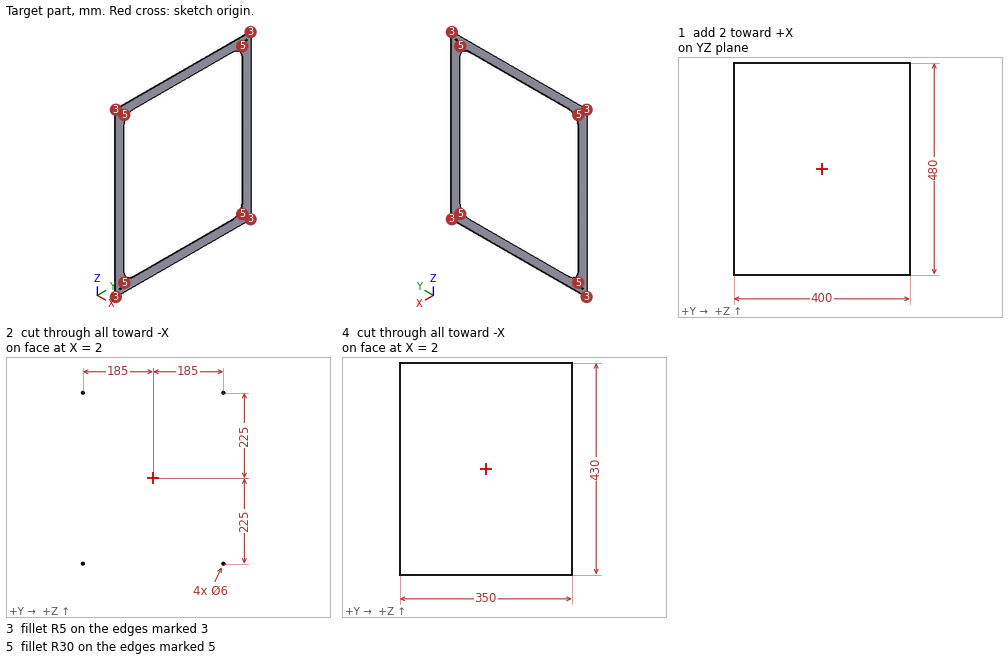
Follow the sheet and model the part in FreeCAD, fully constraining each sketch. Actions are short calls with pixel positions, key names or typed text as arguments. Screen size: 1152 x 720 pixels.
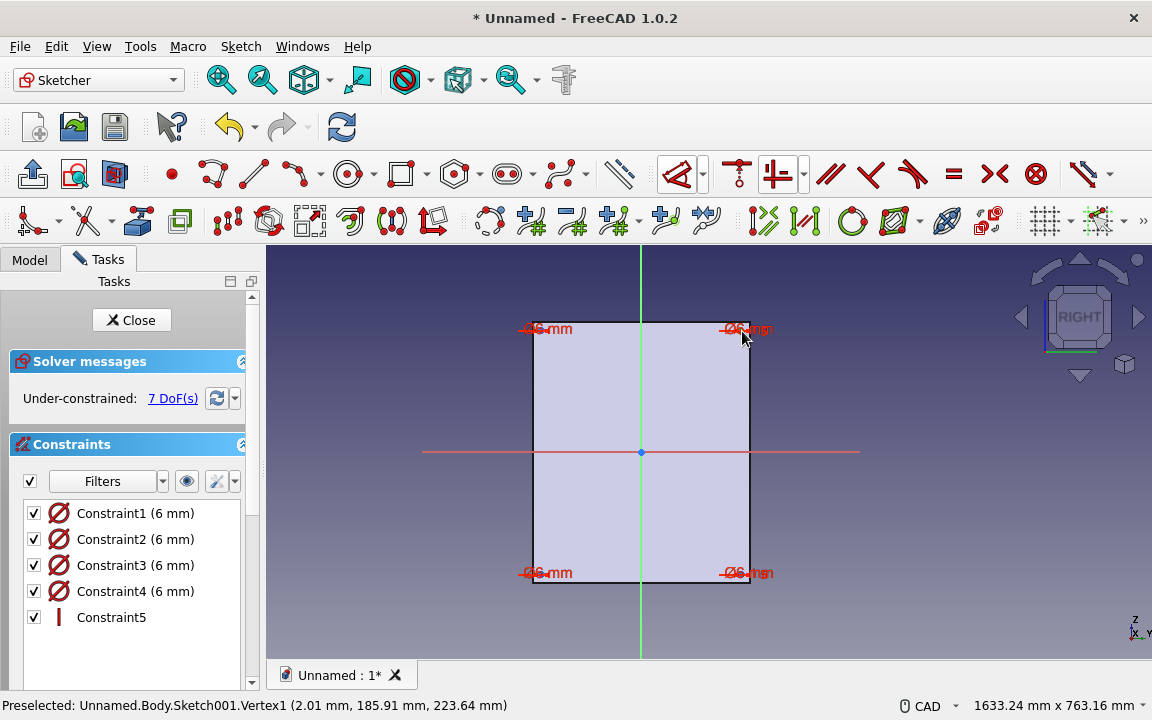
click(541, 331)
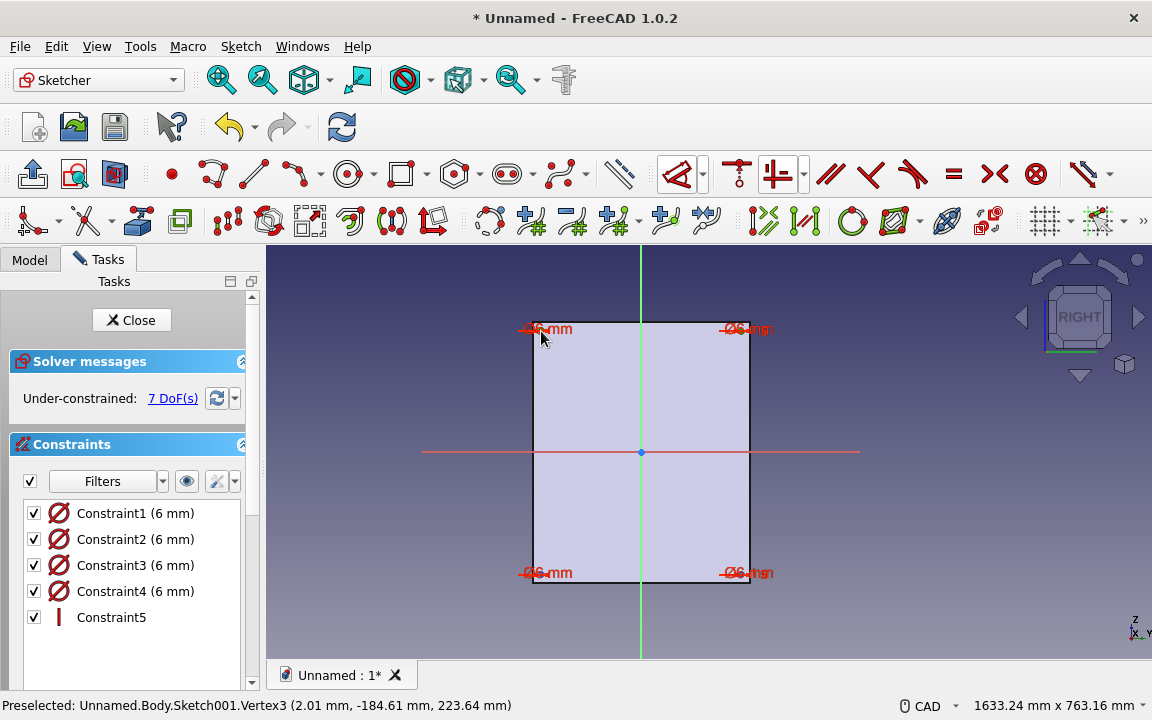
click(804, 174)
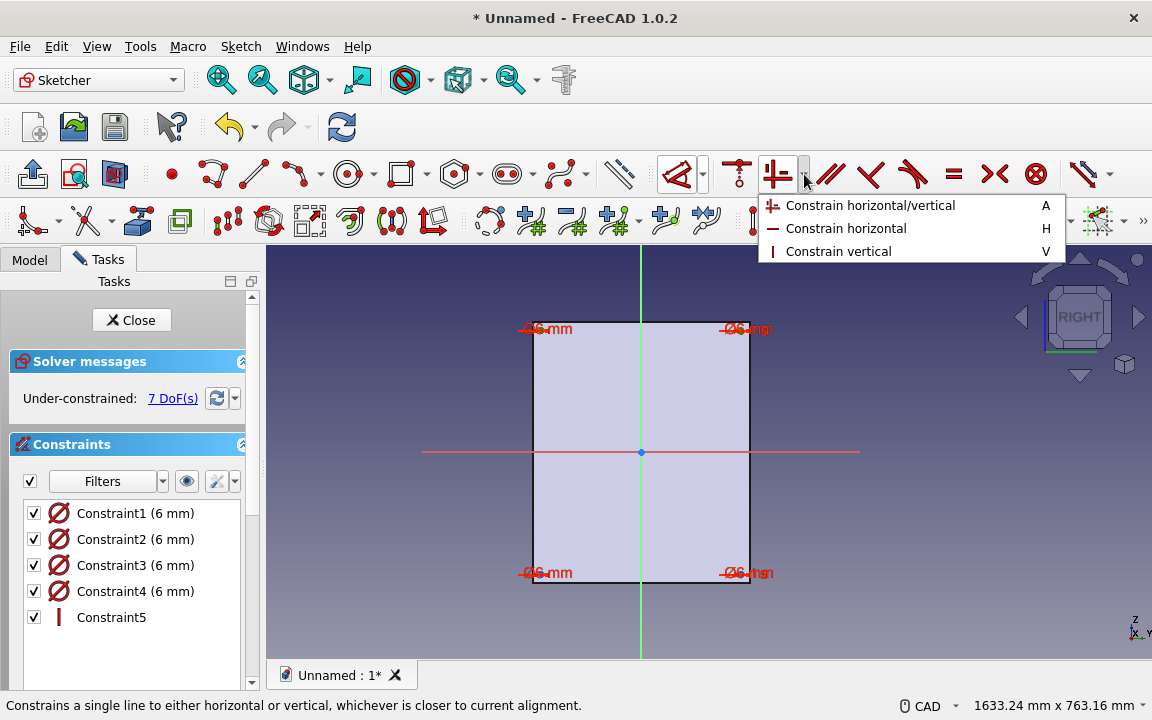
click(912, 228)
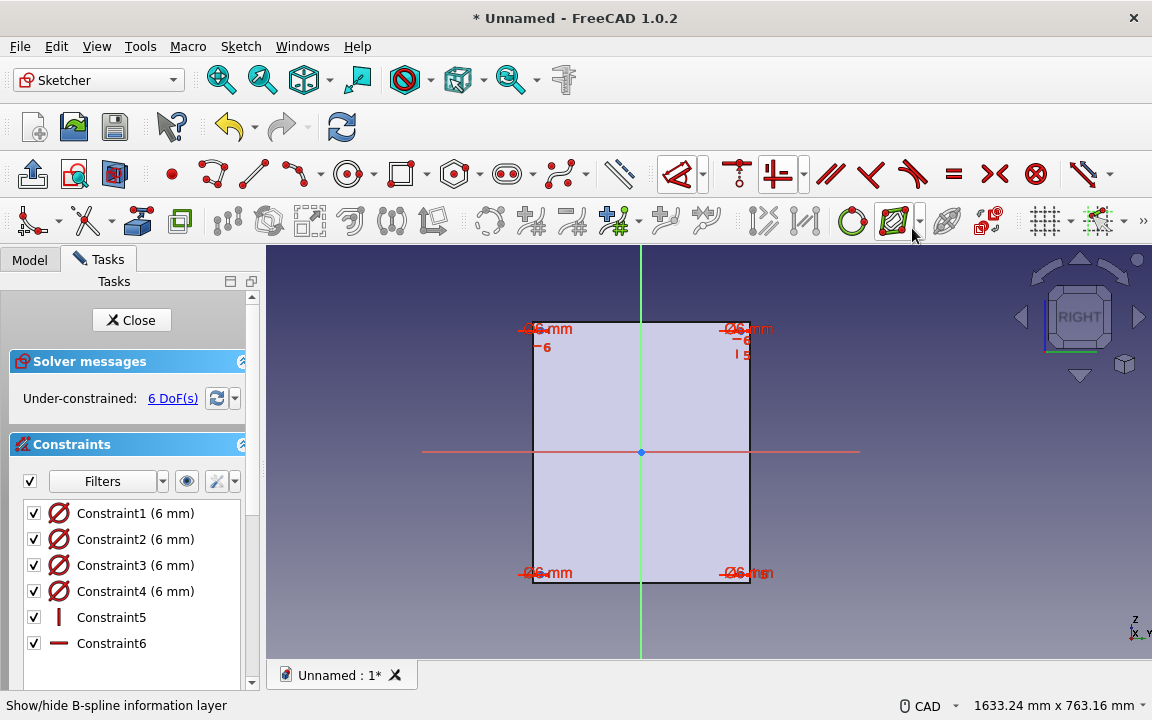
click(541, 331)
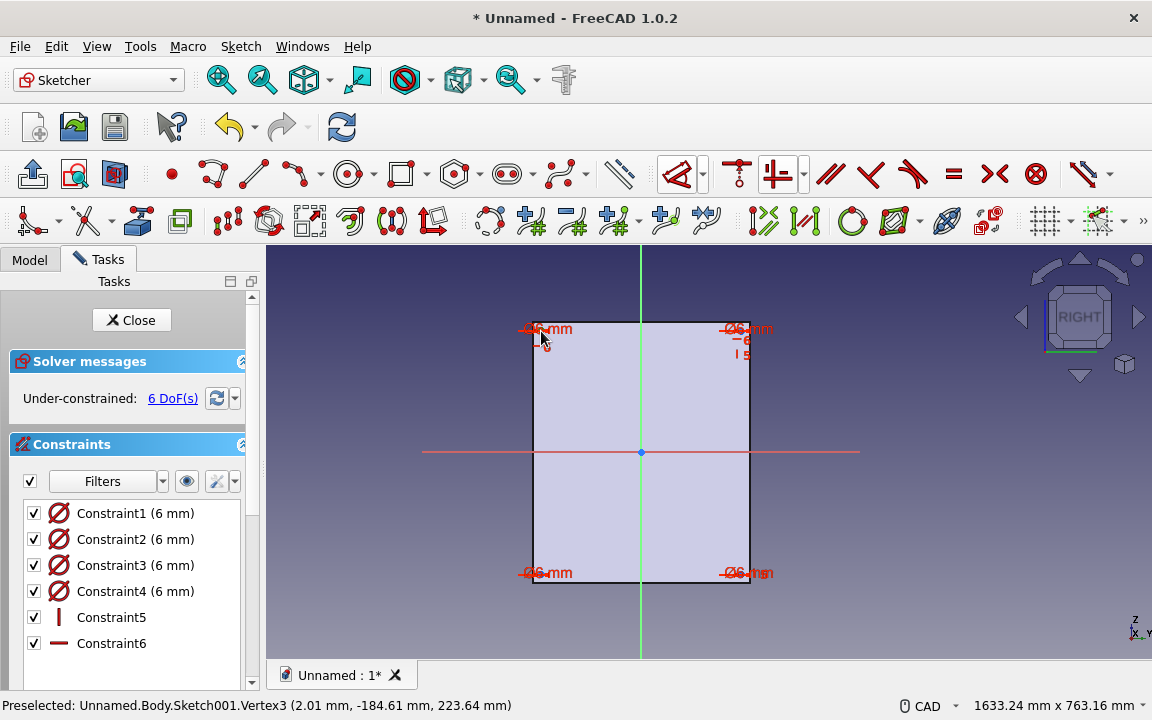
click(541, 575)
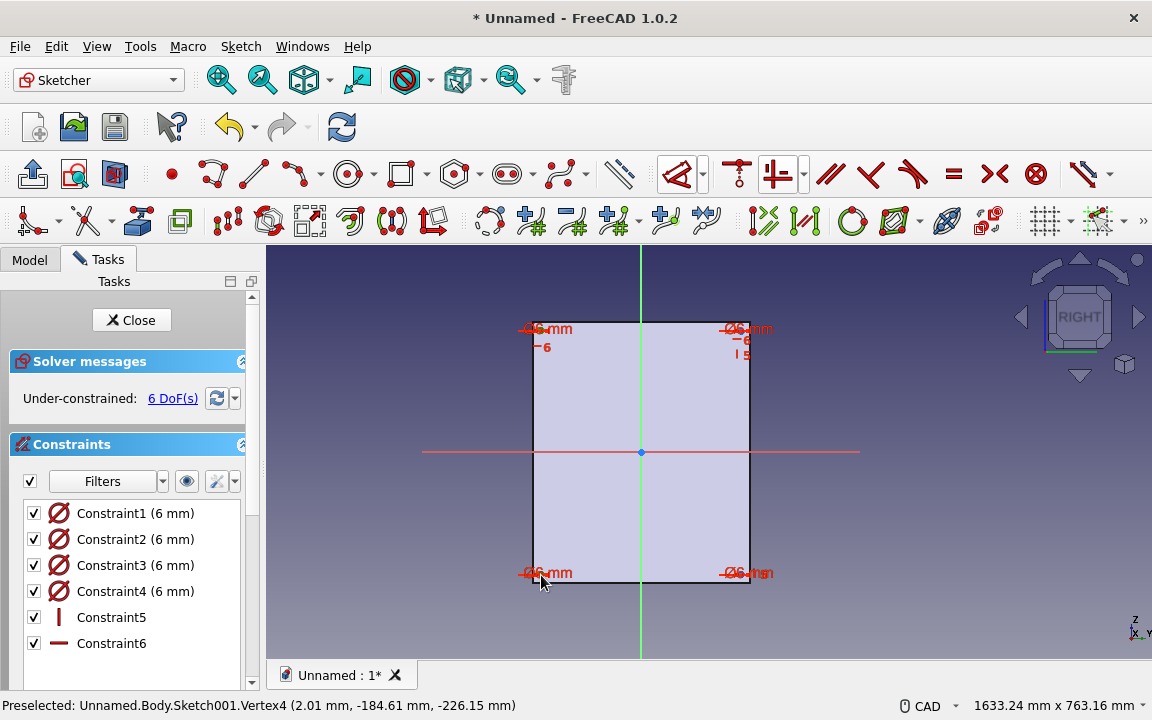
key(v)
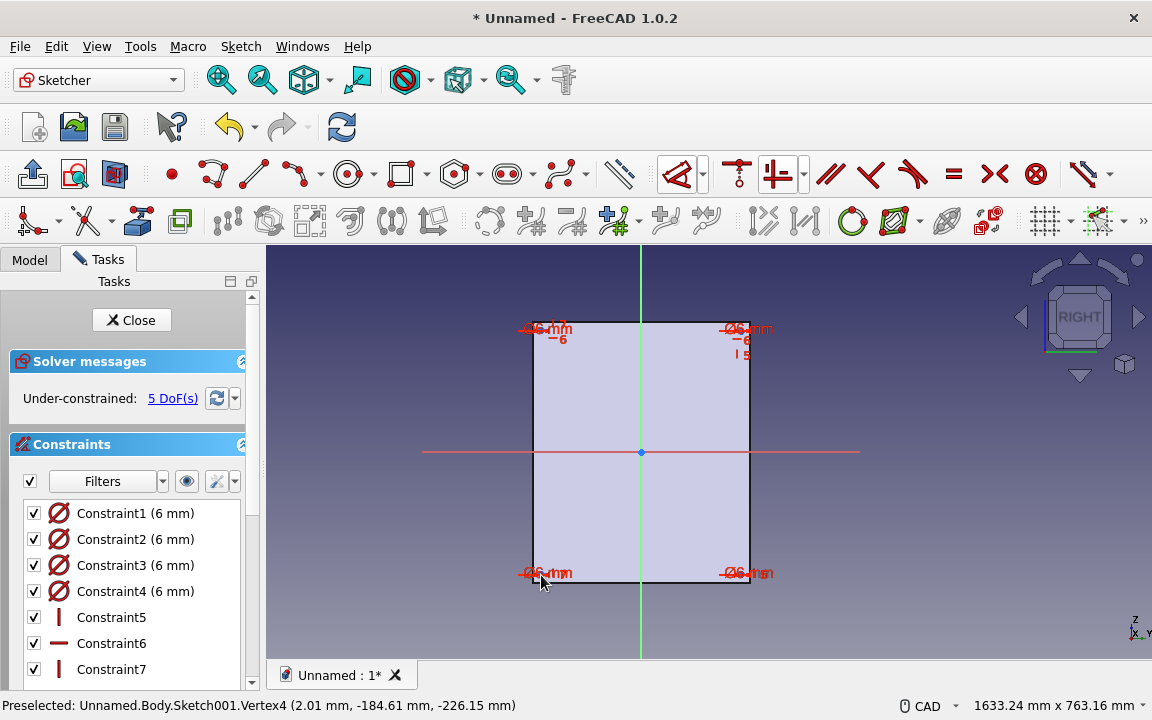
click(742, 575)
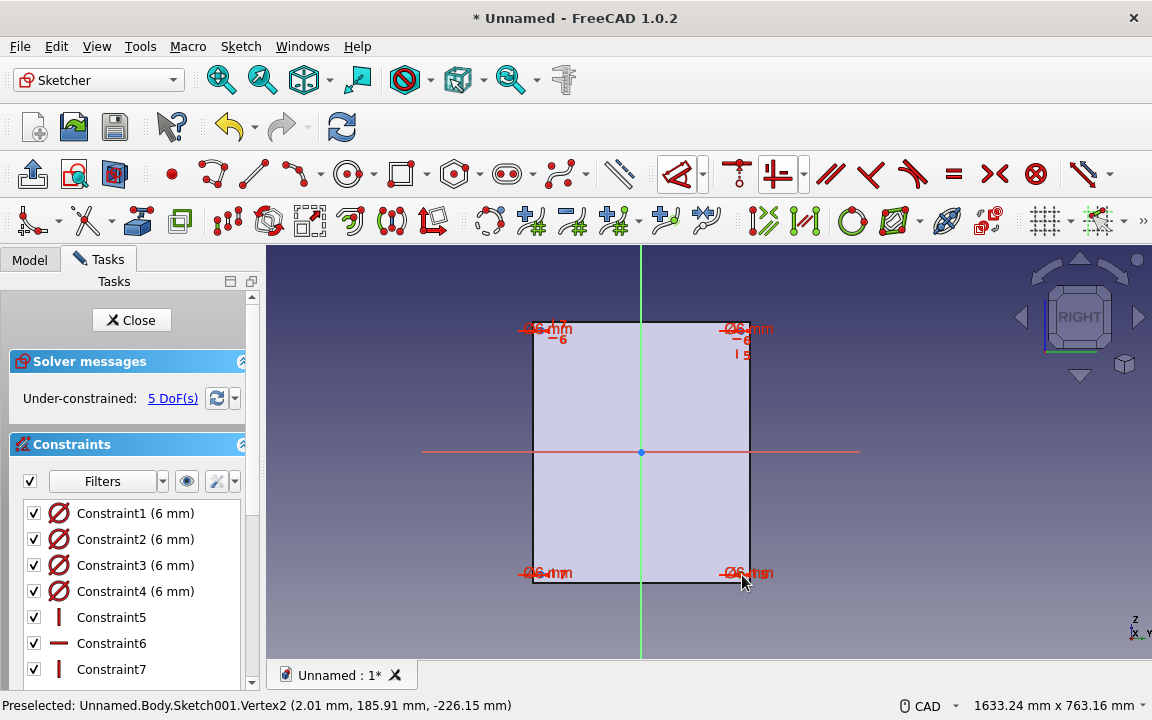
click(541, 575)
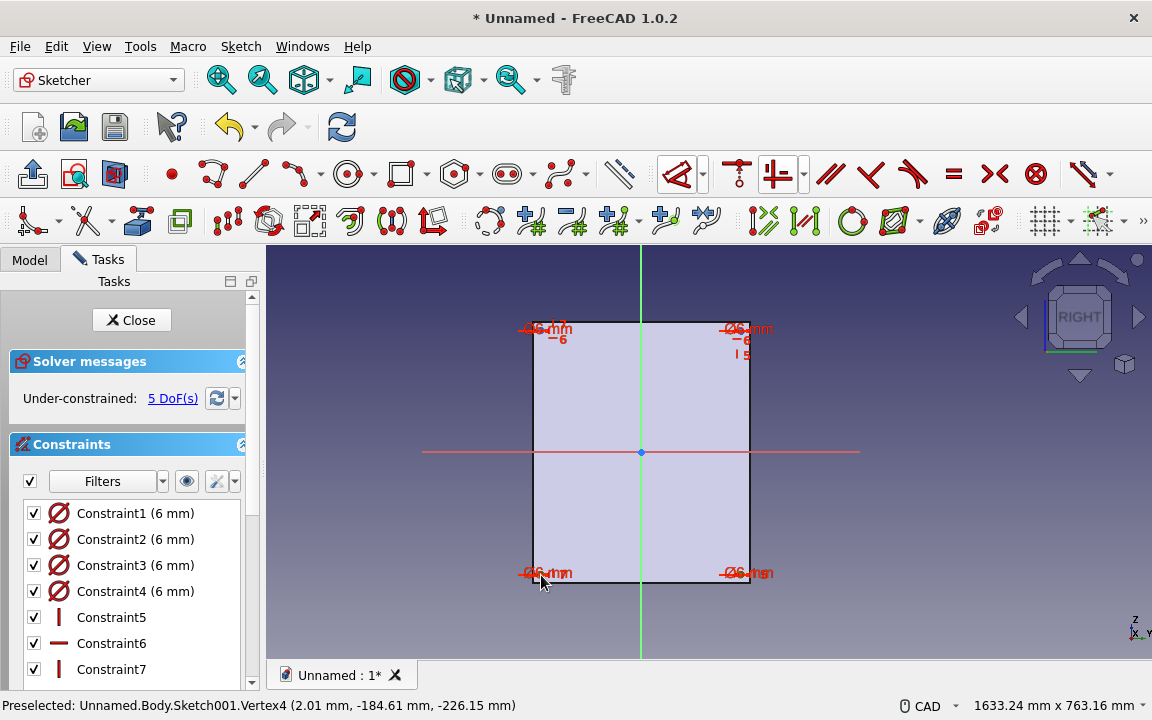
key(h)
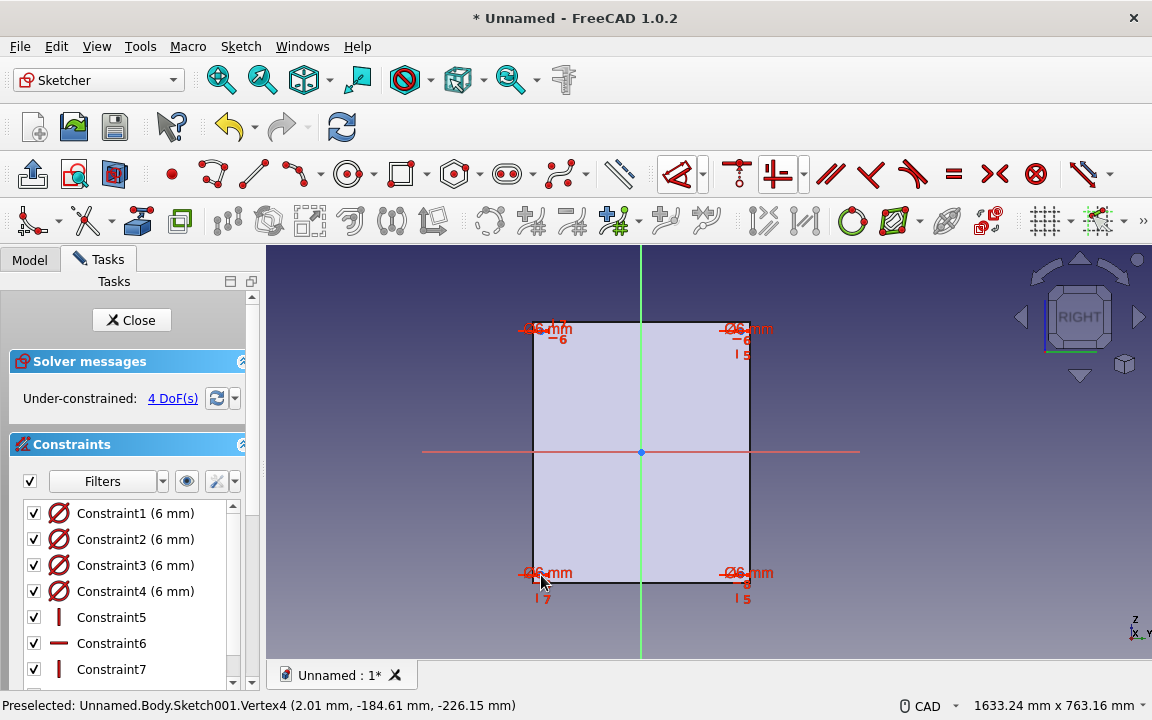
key(d)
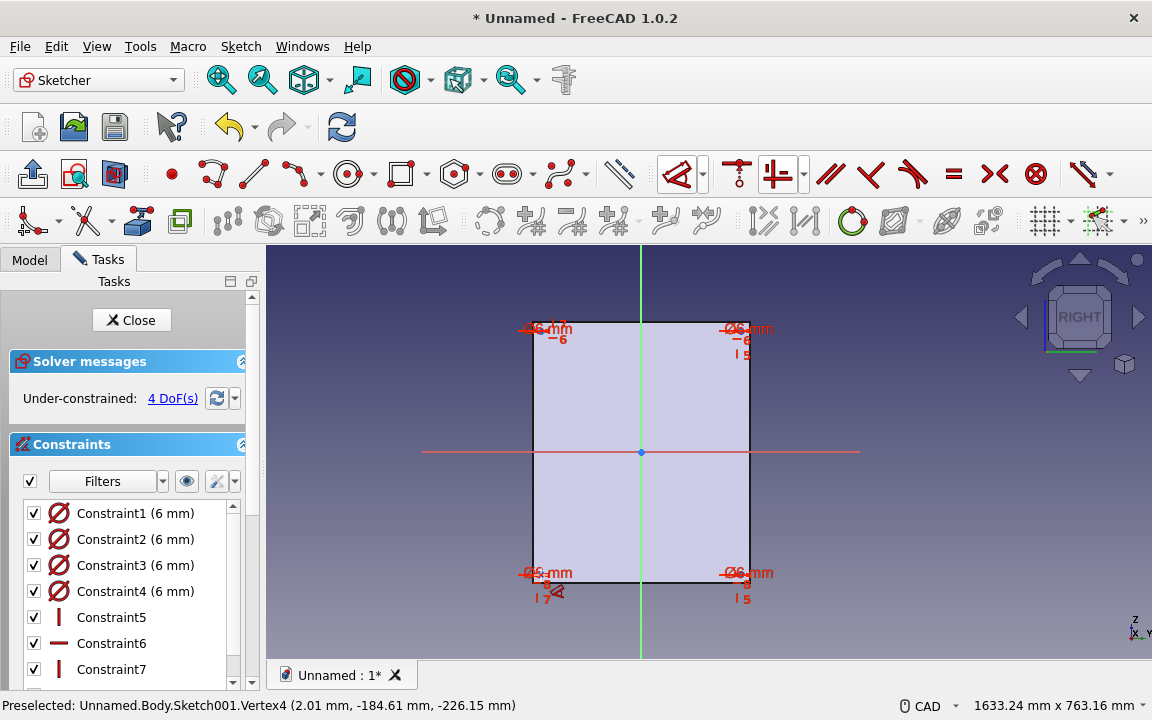
click(742, 331)
click(692, 297)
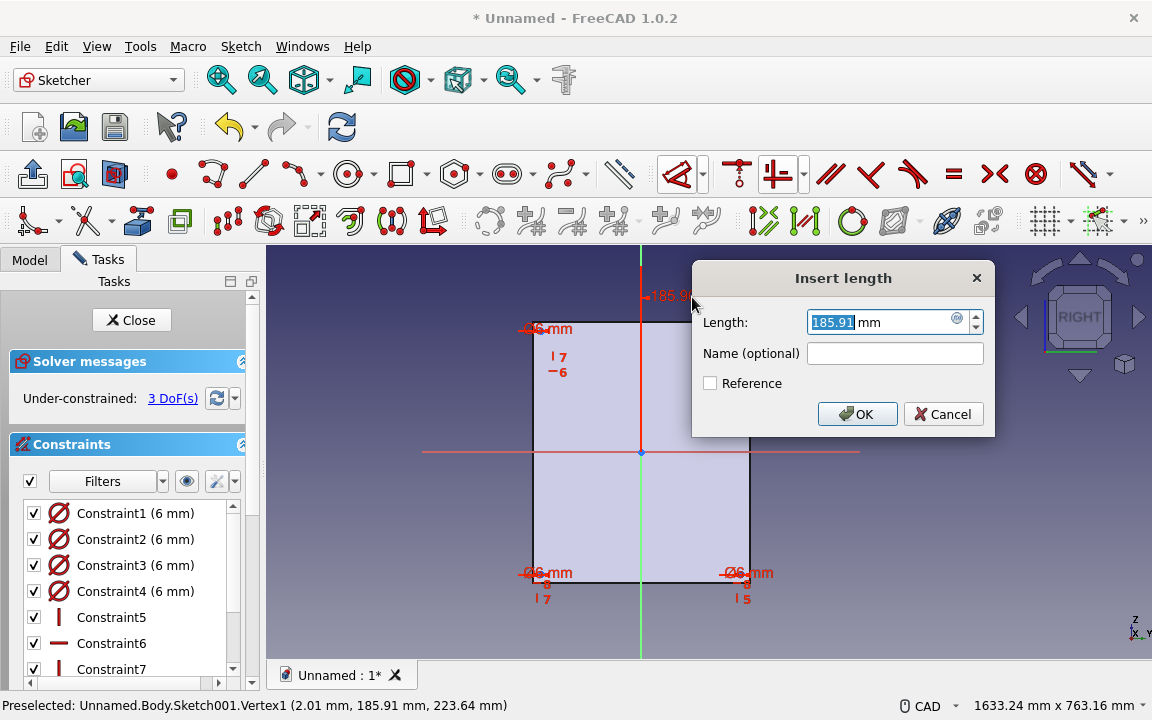
text(185)
key(Return)